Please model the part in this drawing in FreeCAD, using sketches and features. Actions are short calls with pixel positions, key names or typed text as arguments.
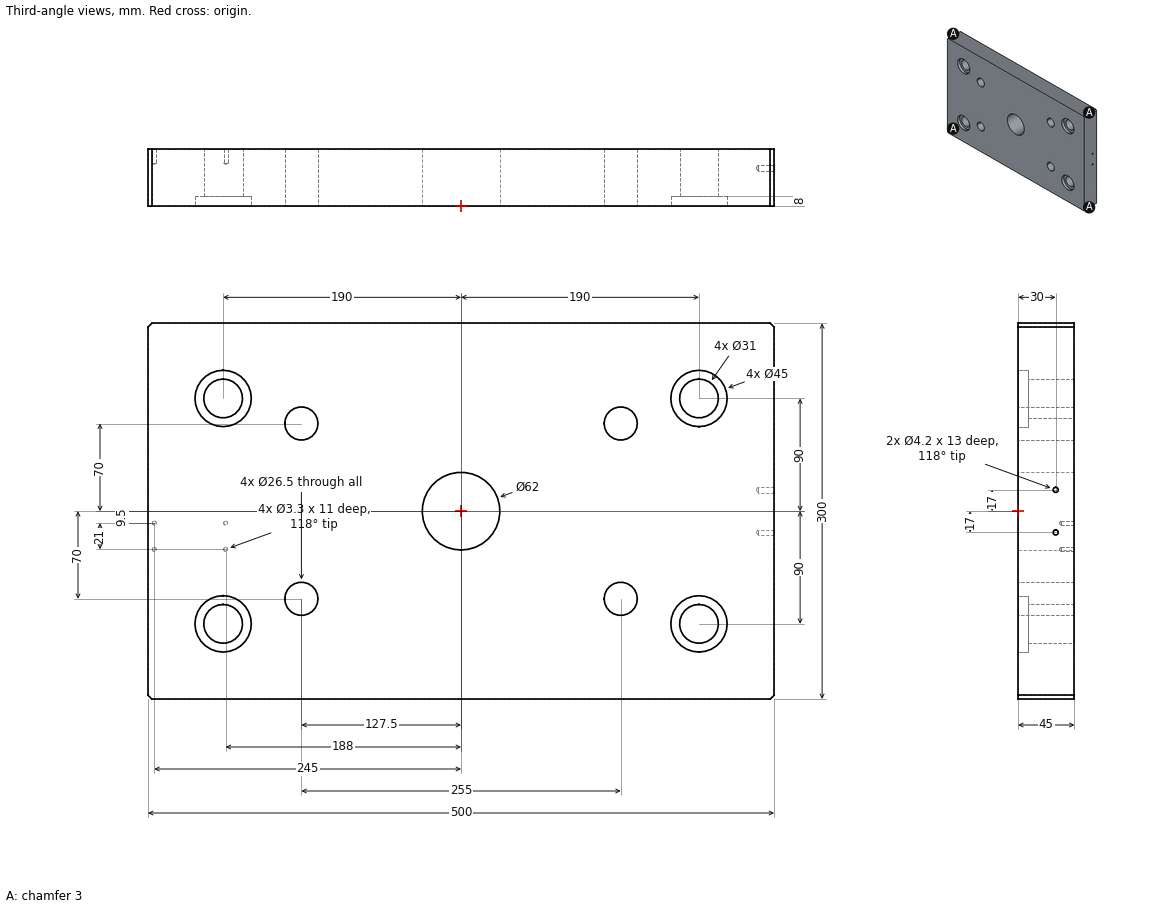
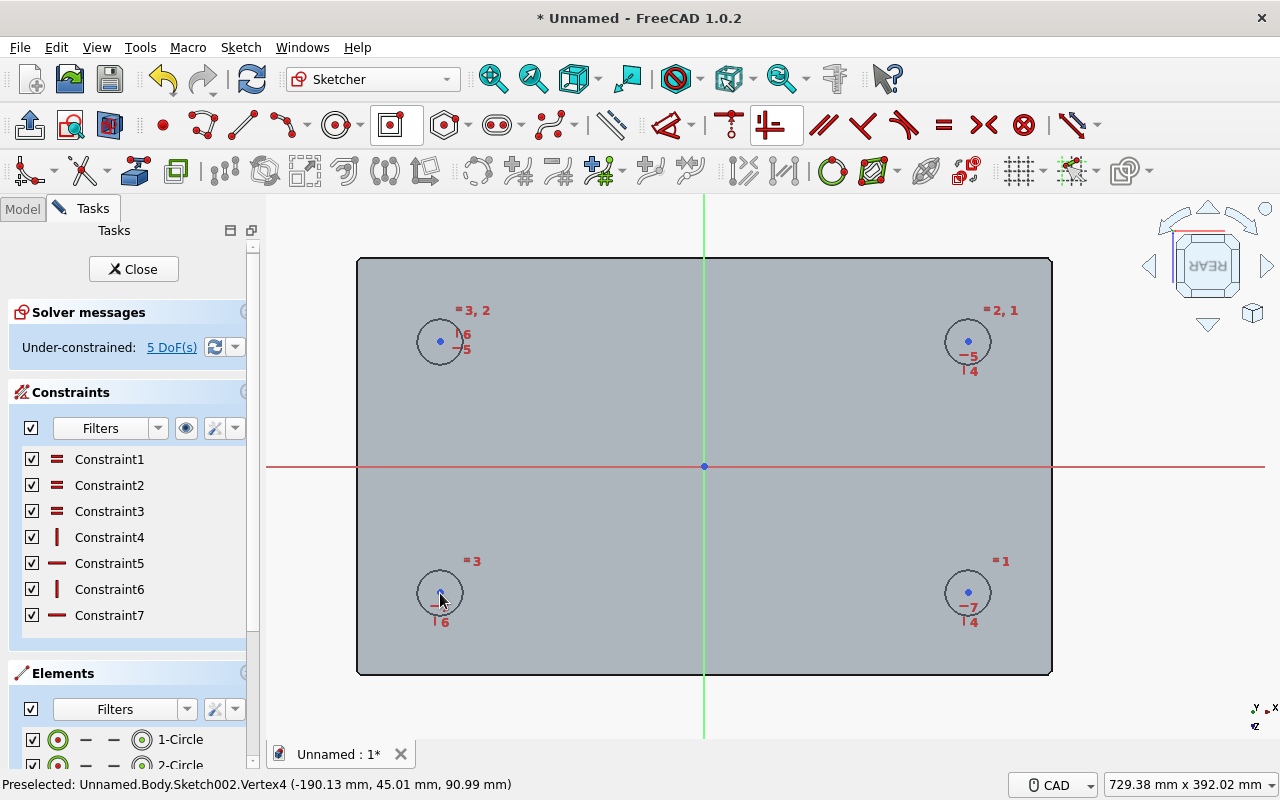
click(666, 126)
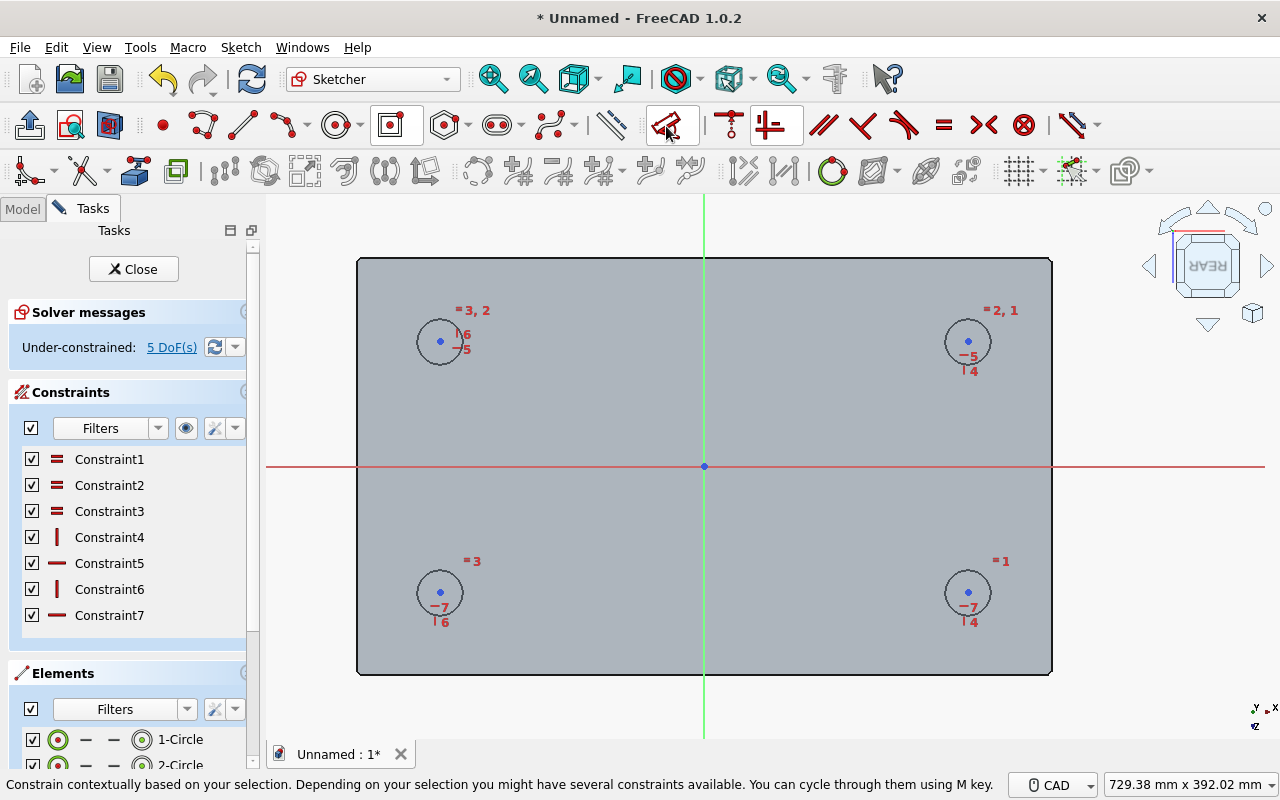
click(984, 577)
click(1007, 554)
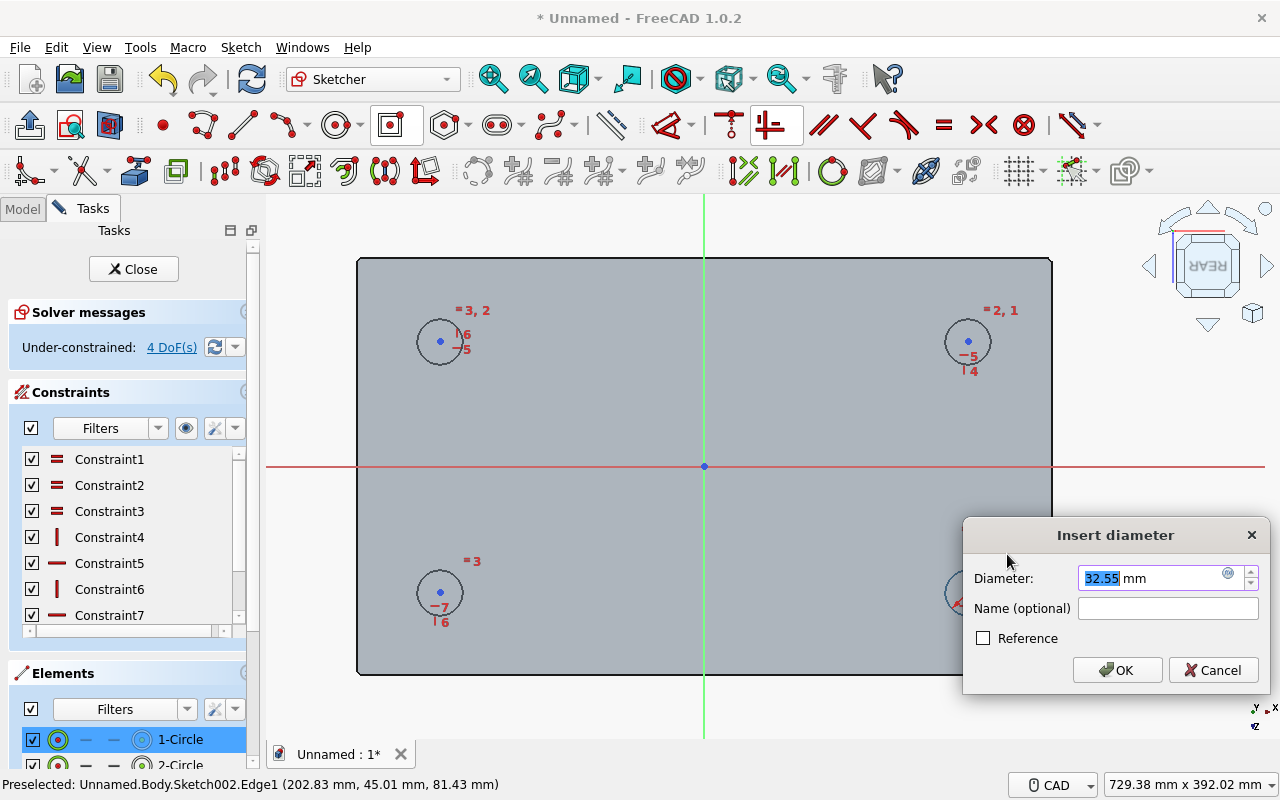
text(31)
key(Return)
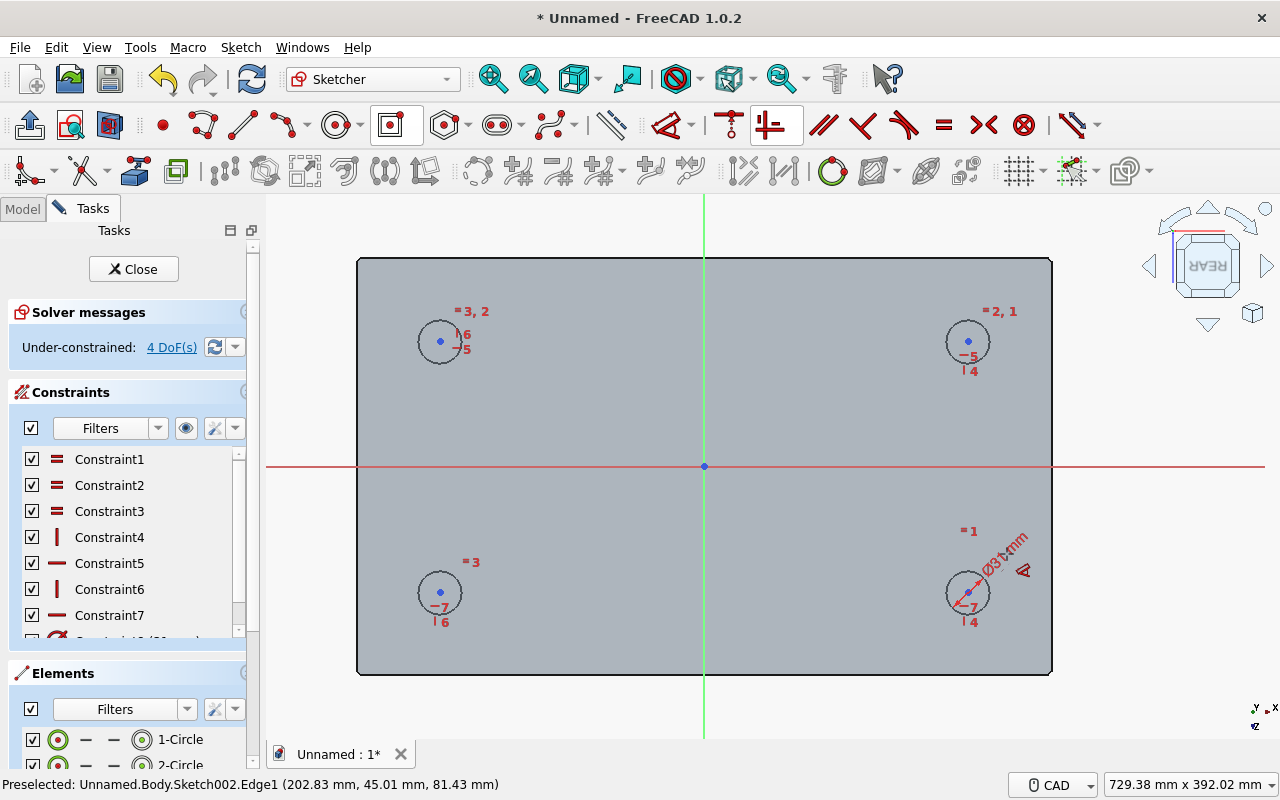
click(968, 593)
click(1002, 530)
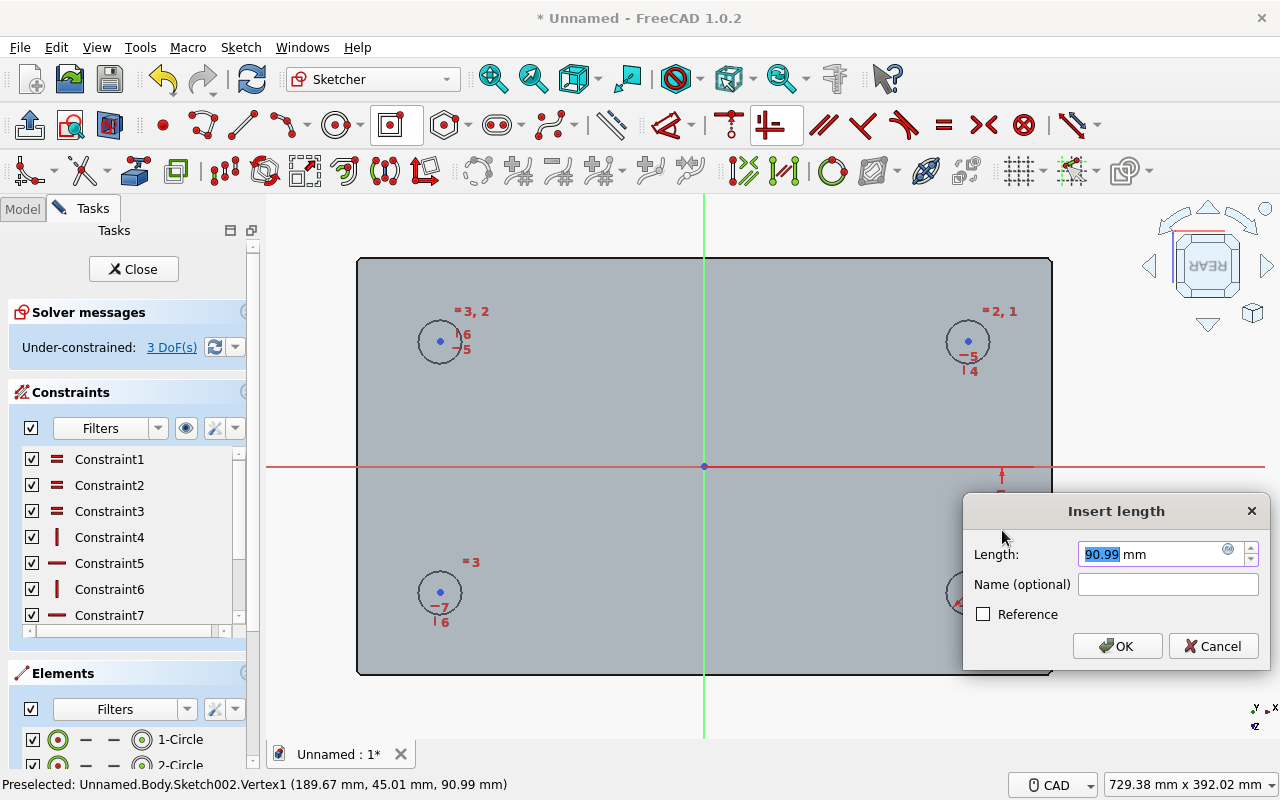
text(90)
key(Return)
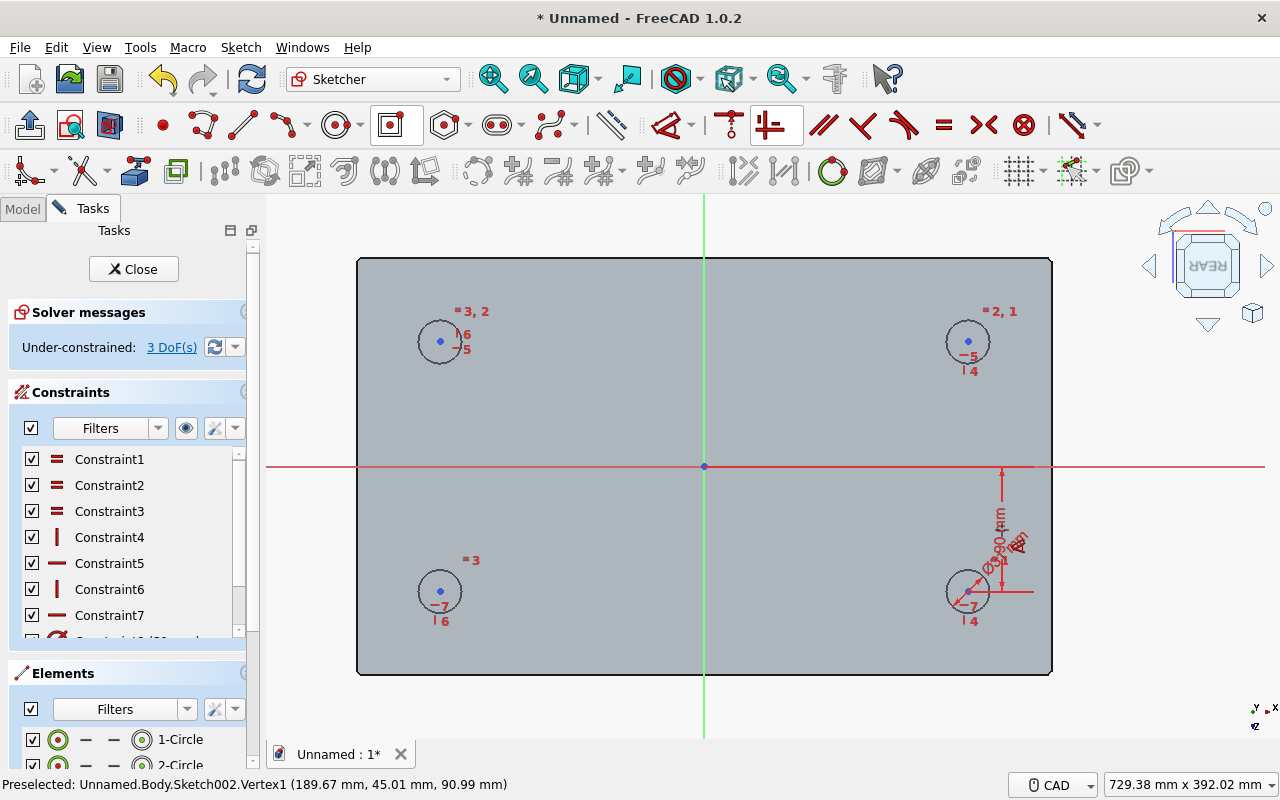
click(968, 342)
click(1002, 404)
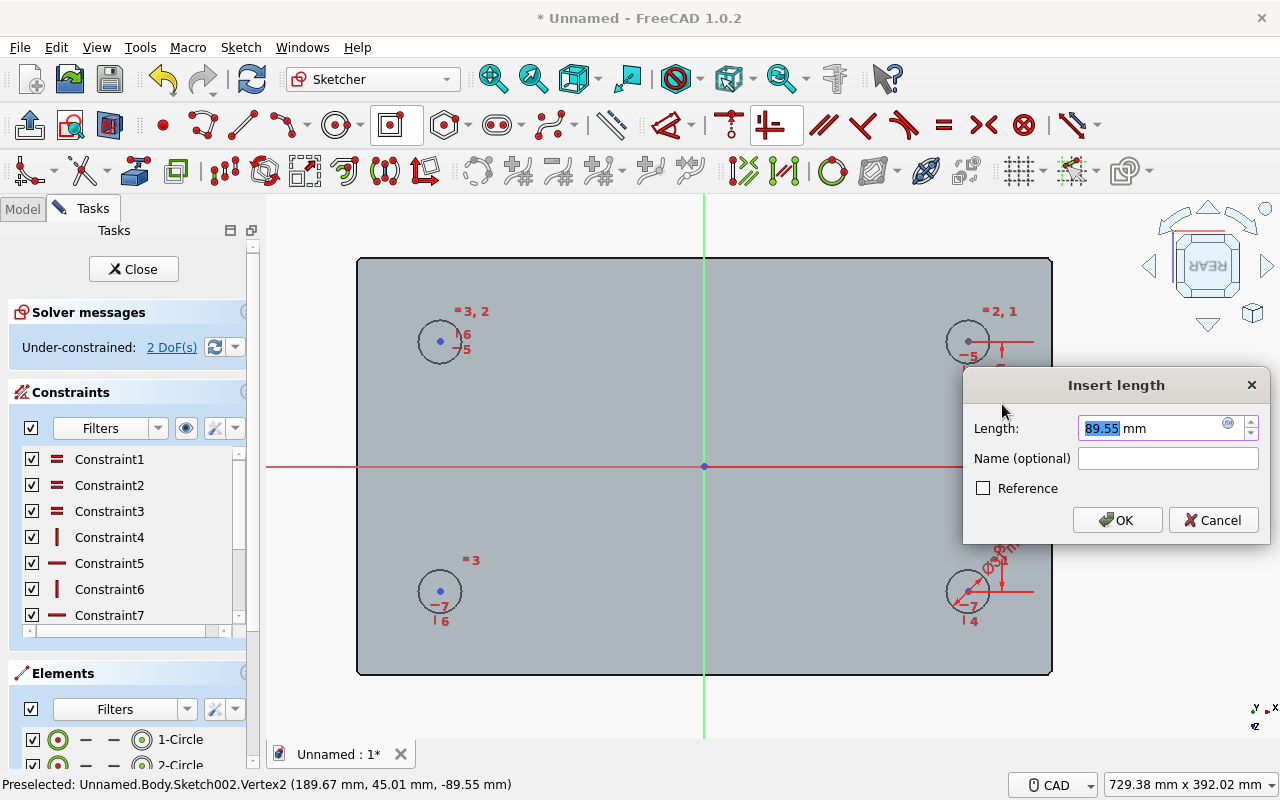
text(90)
key(Return)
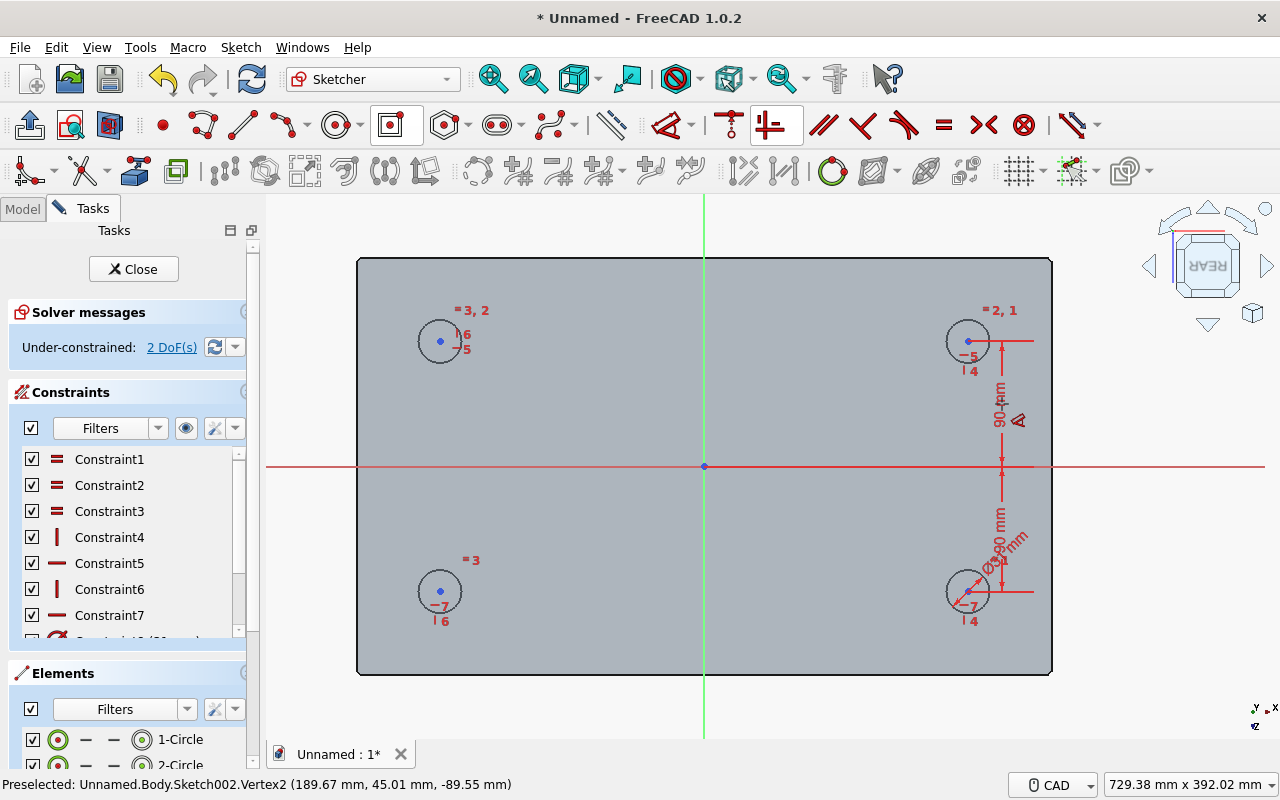
click(968, 592)
click(836, 626)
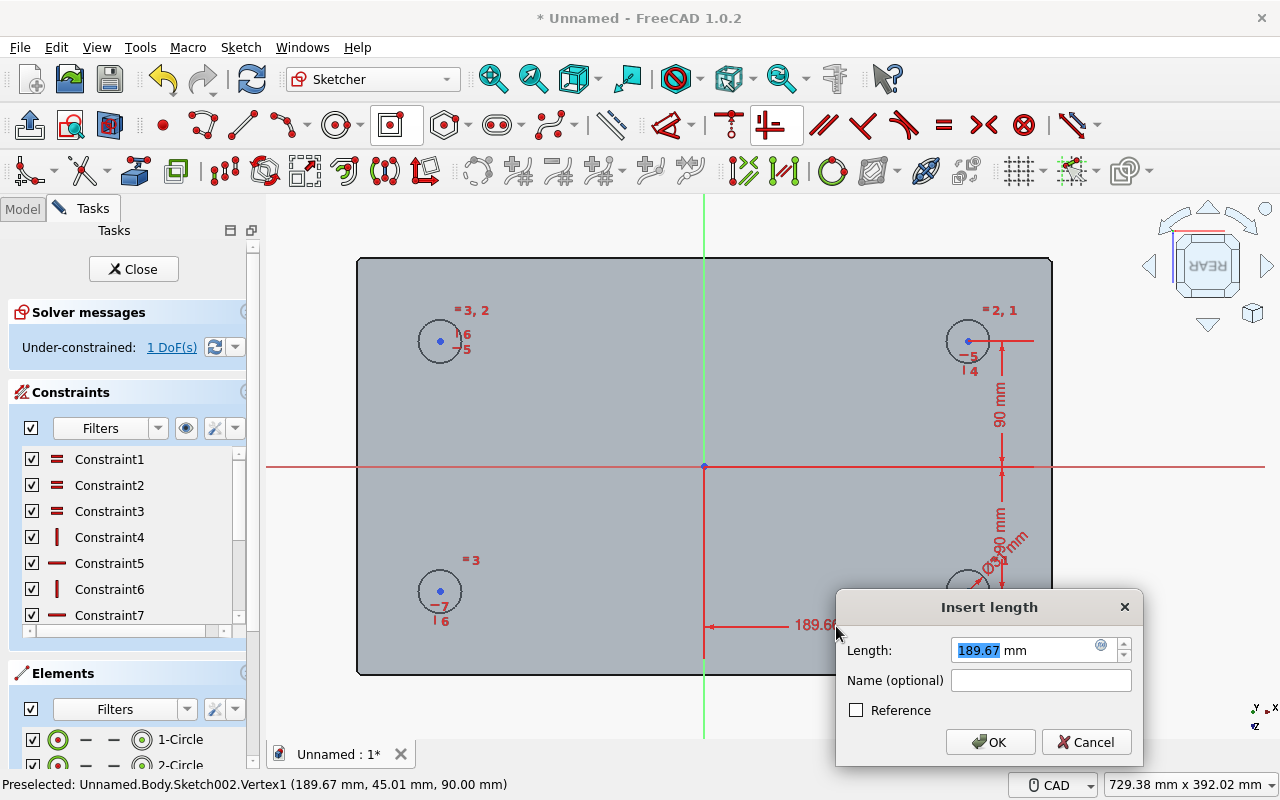
text(190)
key(Return)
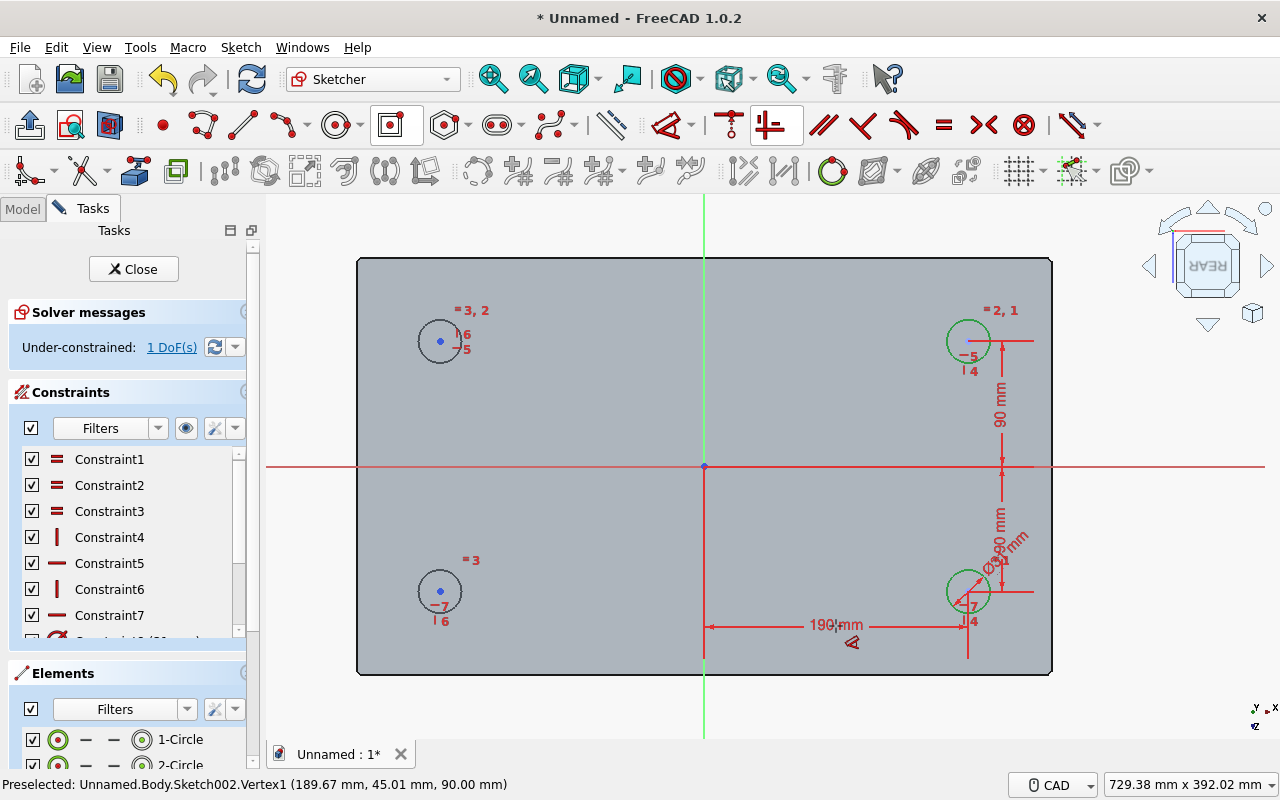
click(440, 341)
click(572, 307)